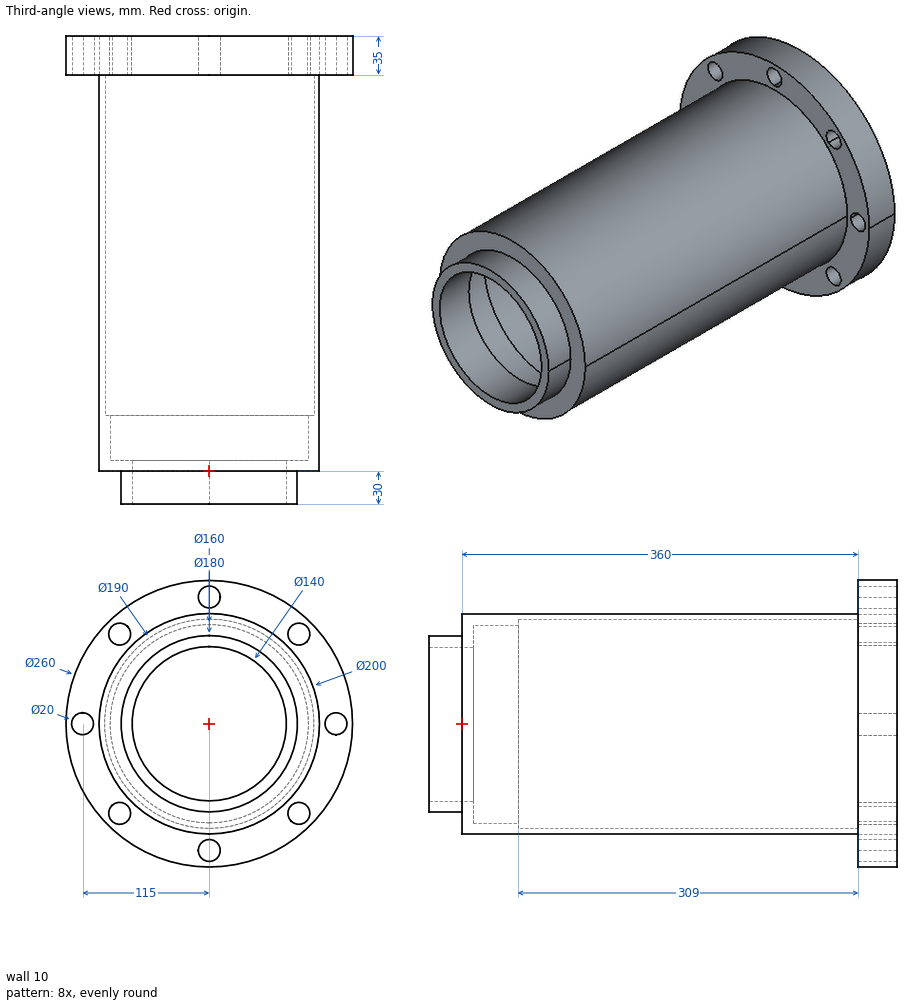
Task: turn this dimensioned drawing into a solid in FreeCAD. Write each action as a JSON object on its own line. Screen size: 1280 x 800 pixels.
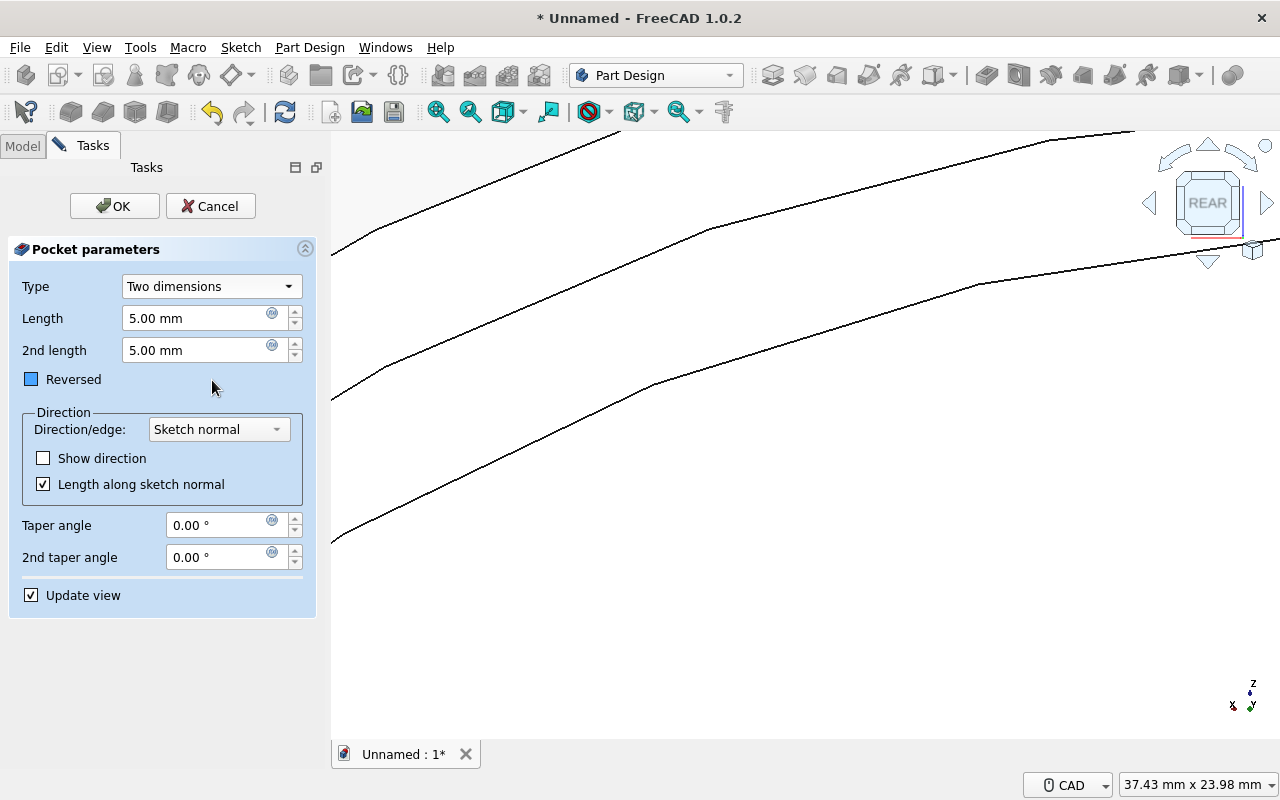
{"action": "triple_click", "coordinate": [204, 318]}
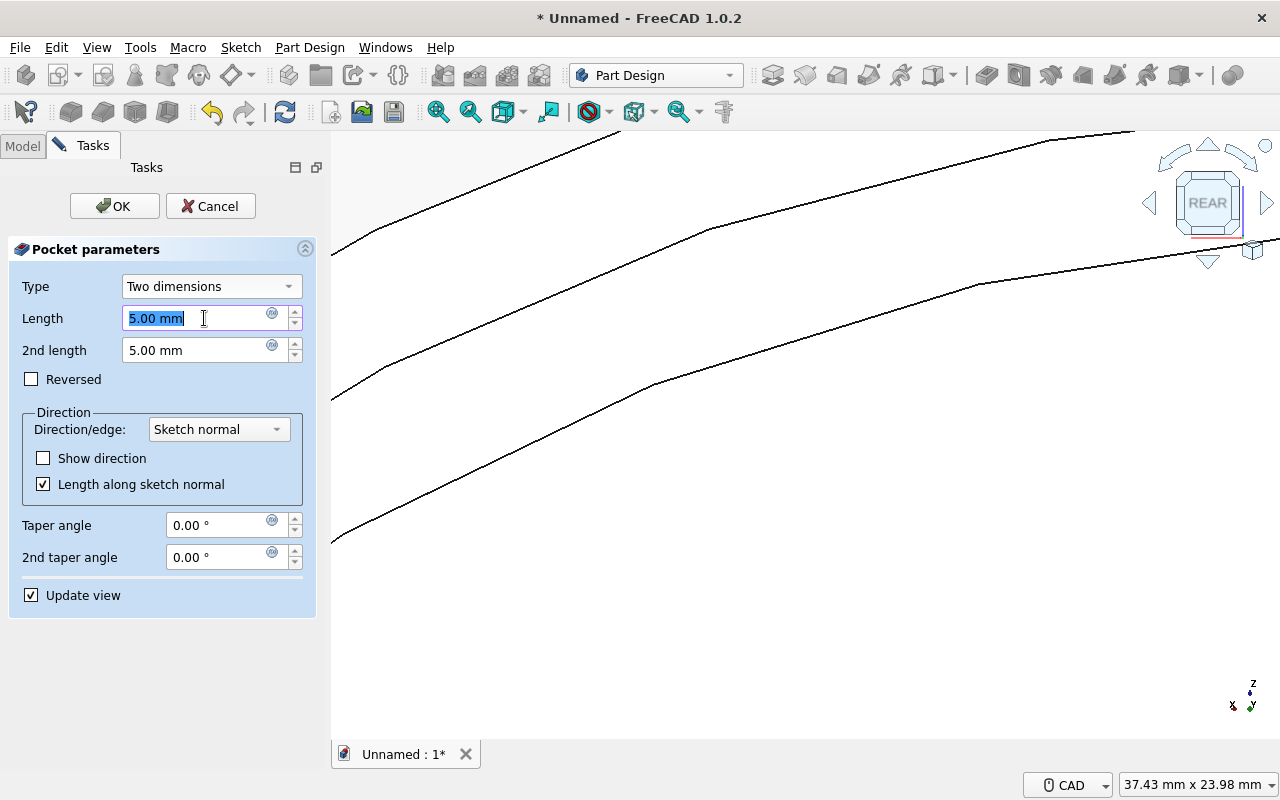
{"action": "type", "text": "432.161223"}
{"action": "key", "text": "Tab"}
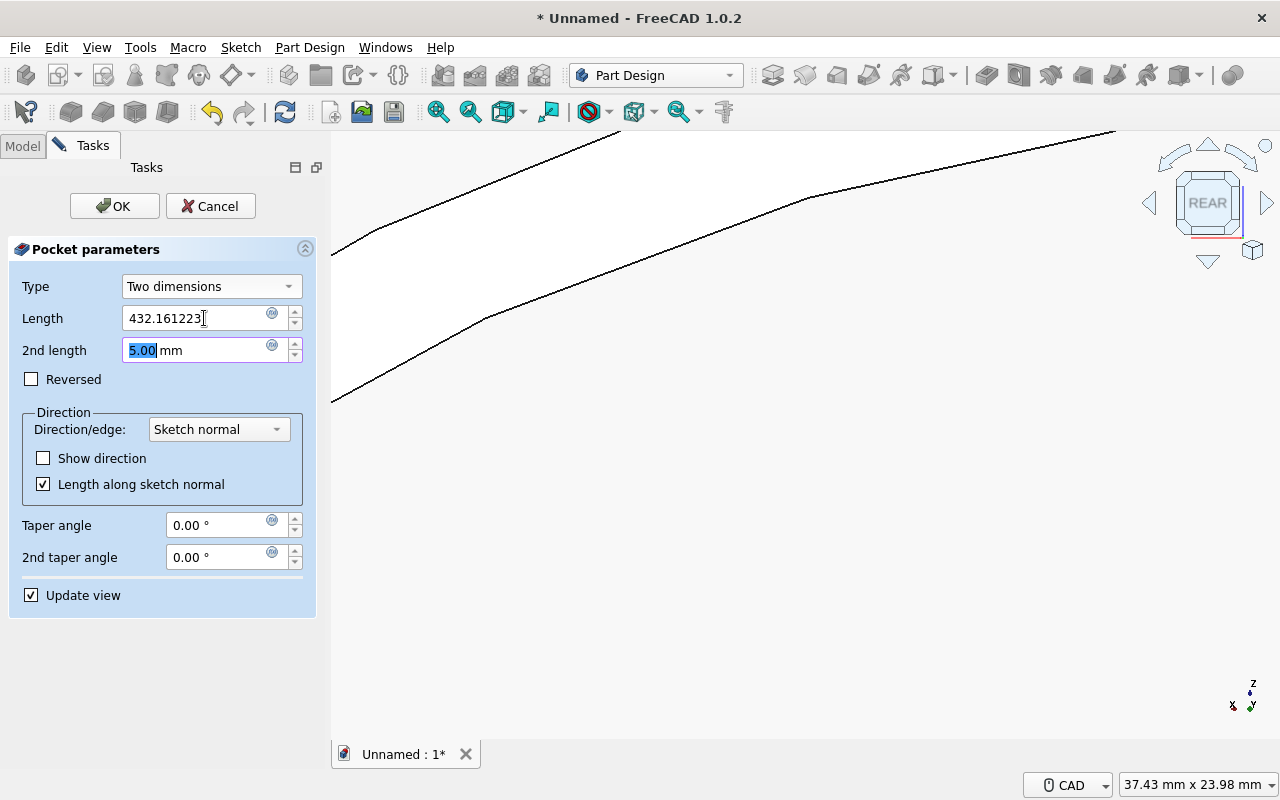
{"action": "type", "text": "309"}
{"action": "key", "text": "Tab"}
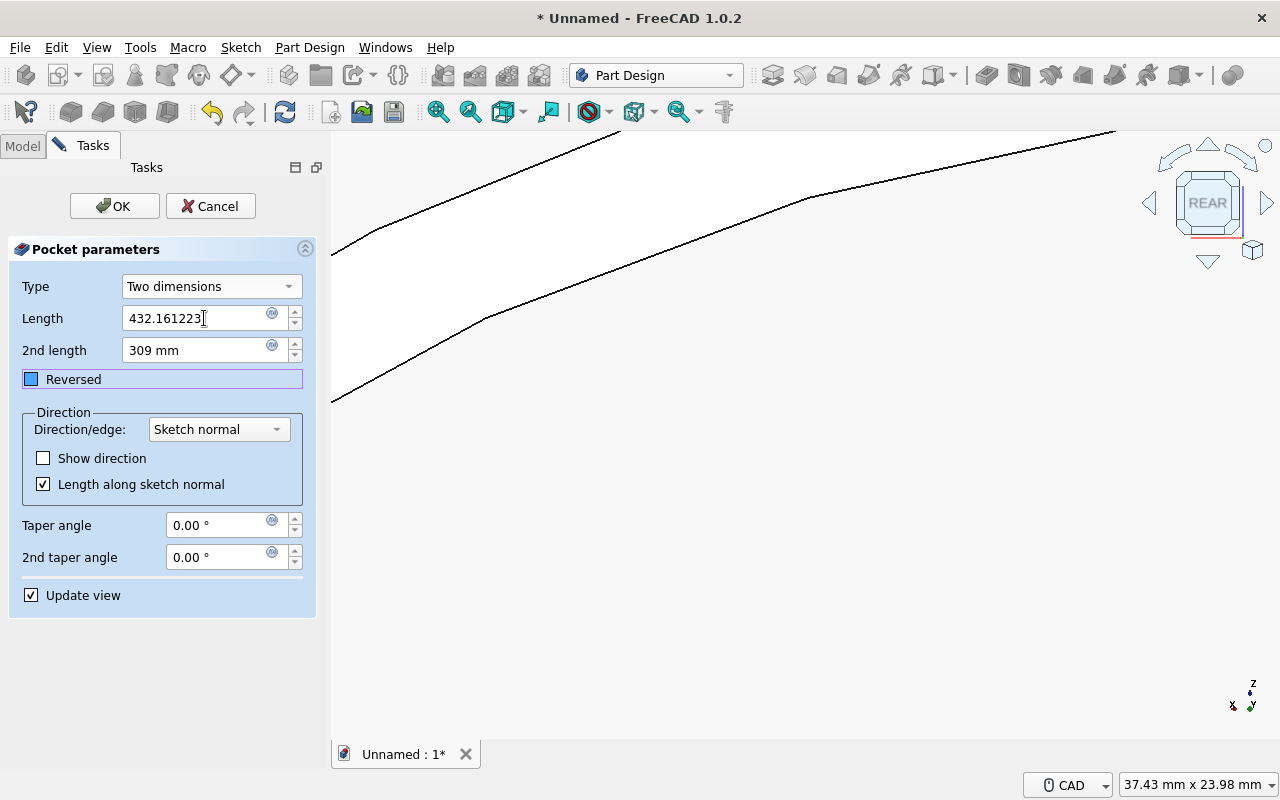
{"action": "left_click", "coordinate": [30, 379]}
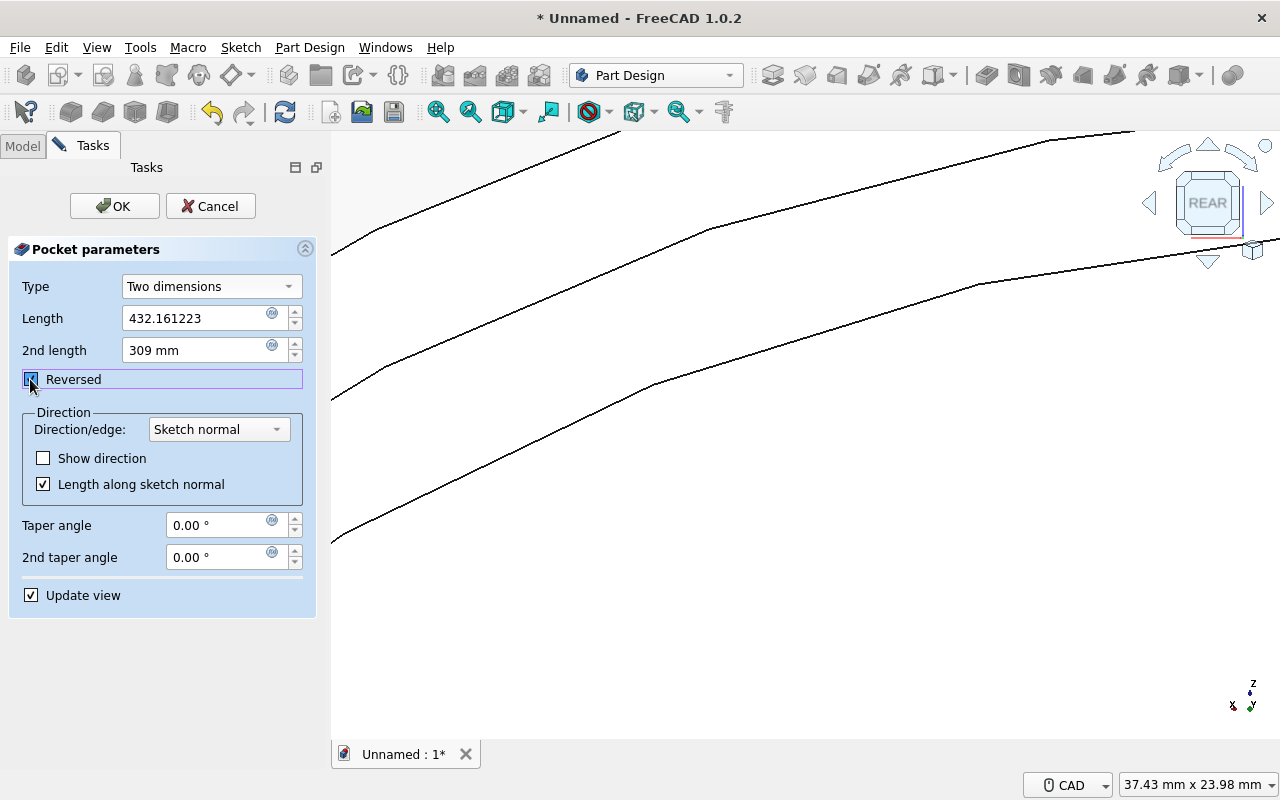
{"action": "left_click", "coordinate": [115, 206]}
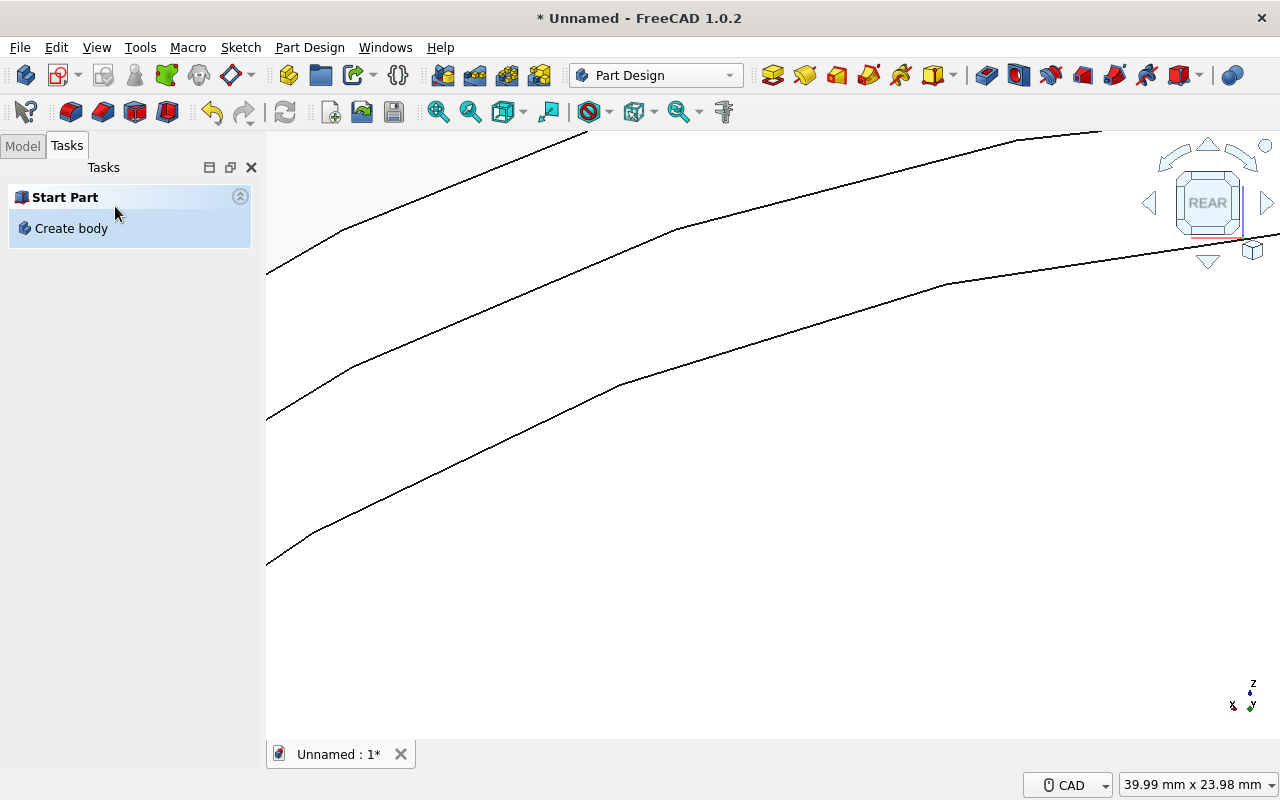
{"action": "key", "text": "v f"}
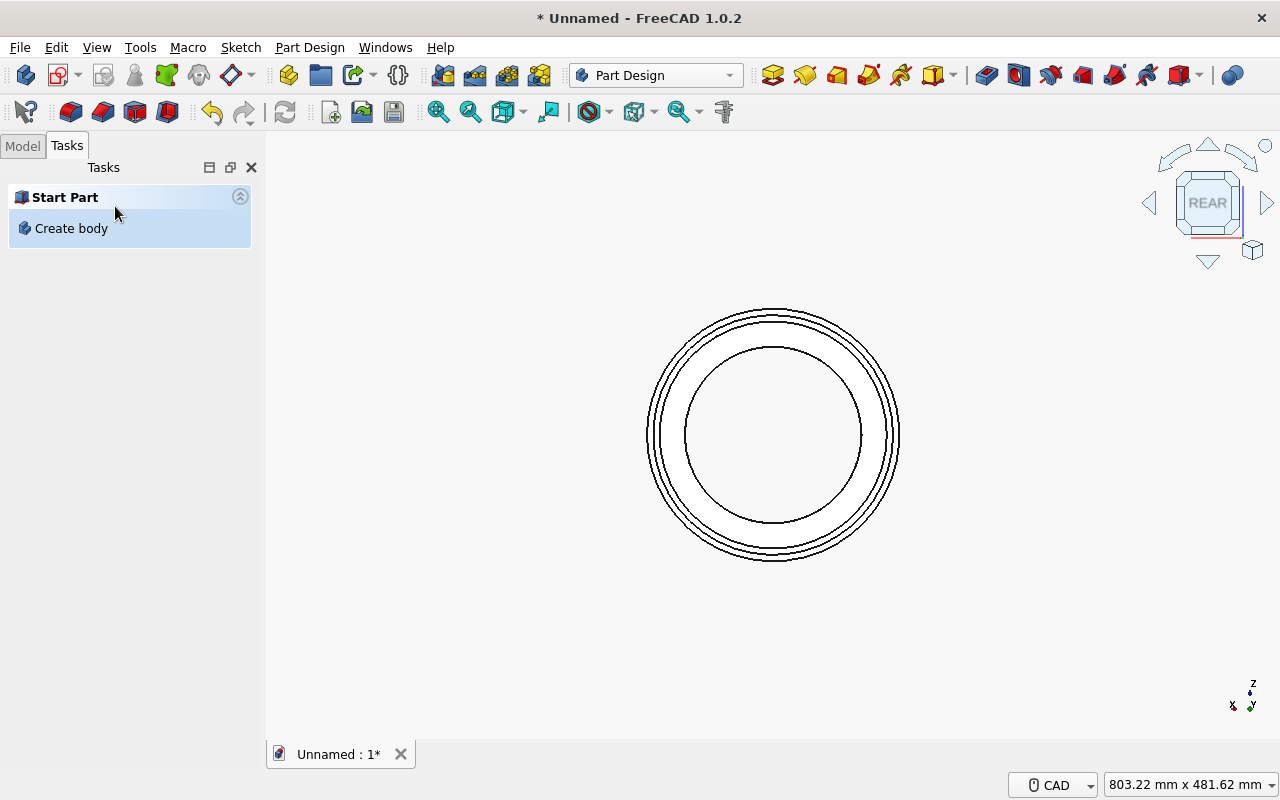
{"action": "left_click", "coordinate": [26, 76]}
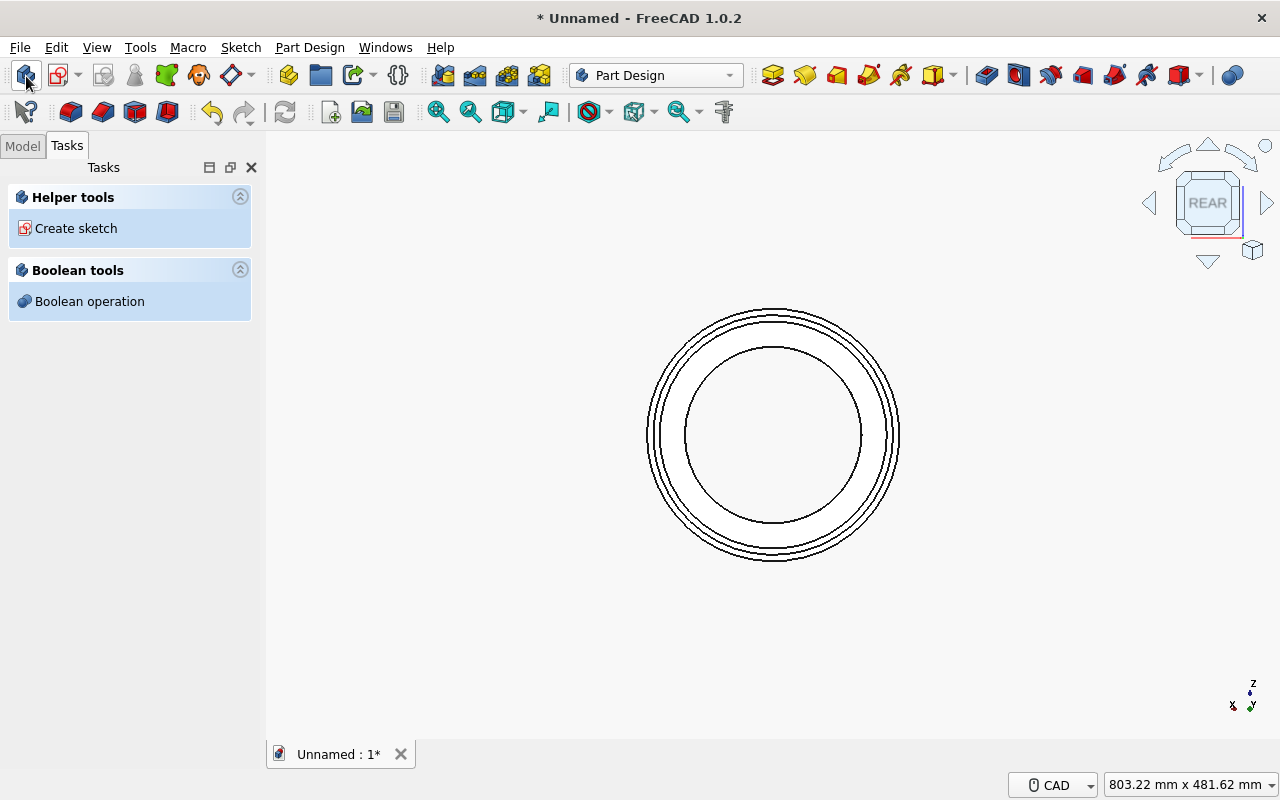
{"action": "left_click", "coordinate": [23, 145]}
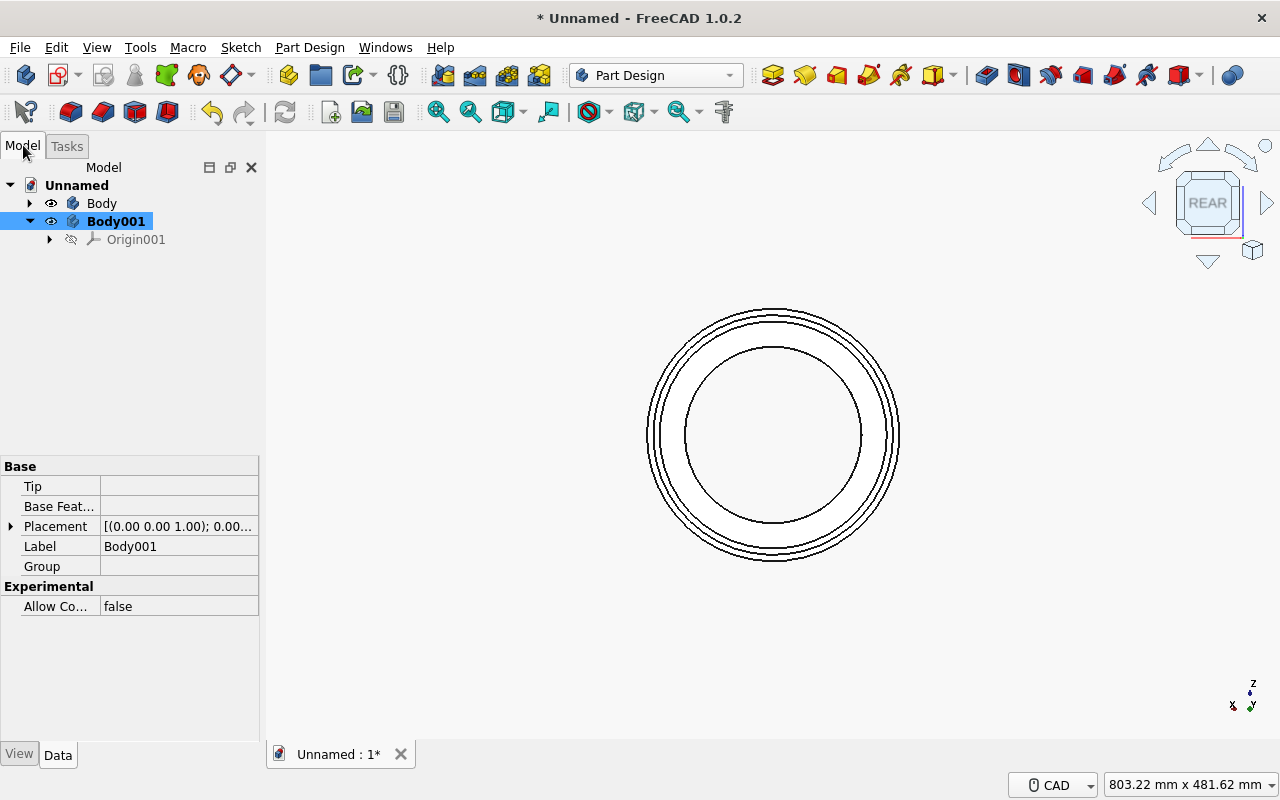
{"action": "left_click", "coordinate": [50, 239]}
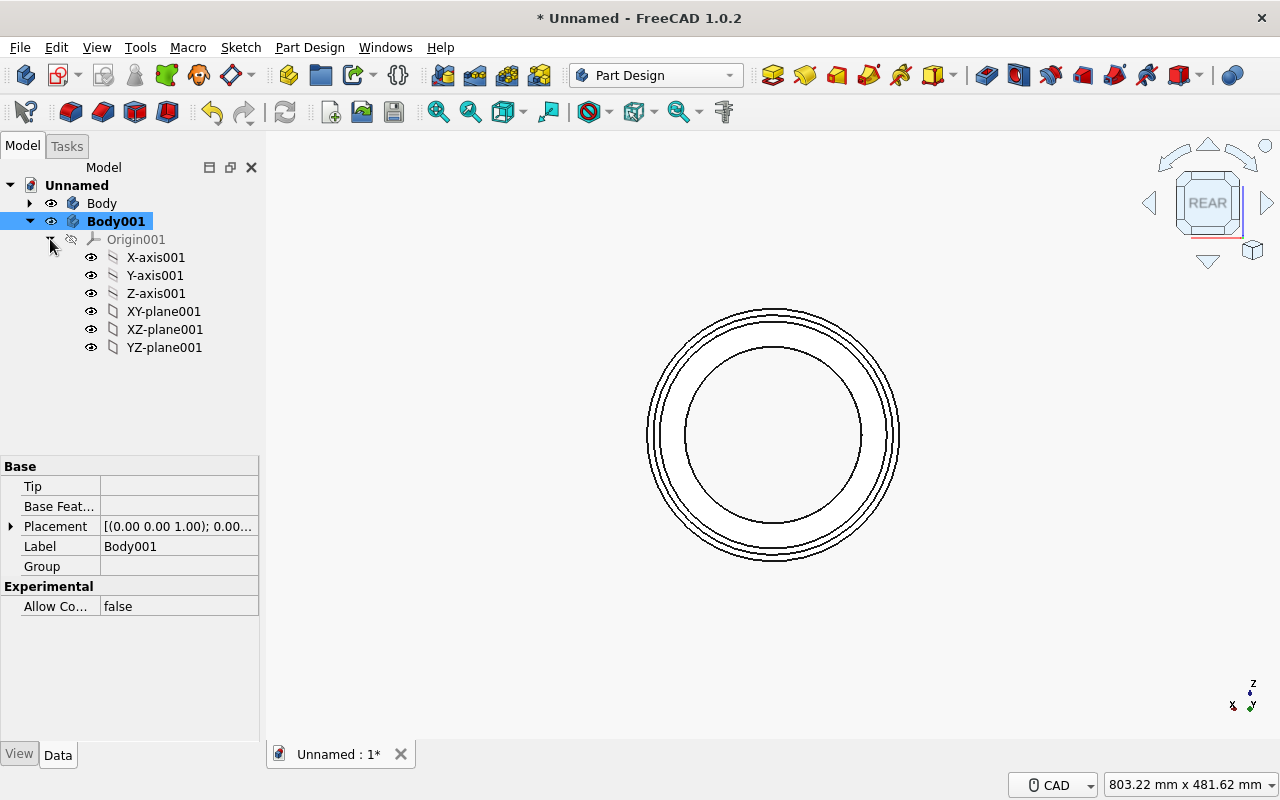
{"action": "left_click", "coordinate": [136, 329]}